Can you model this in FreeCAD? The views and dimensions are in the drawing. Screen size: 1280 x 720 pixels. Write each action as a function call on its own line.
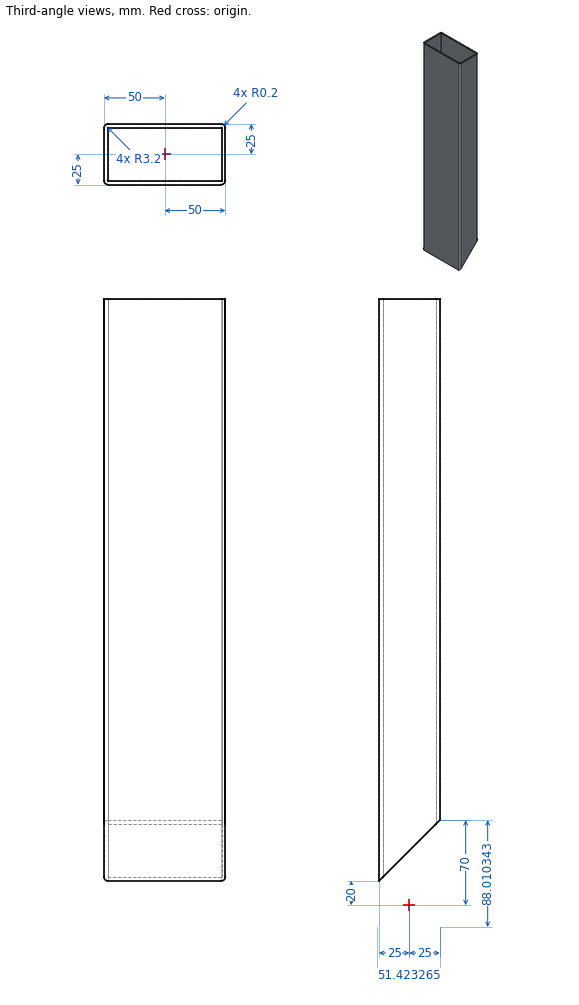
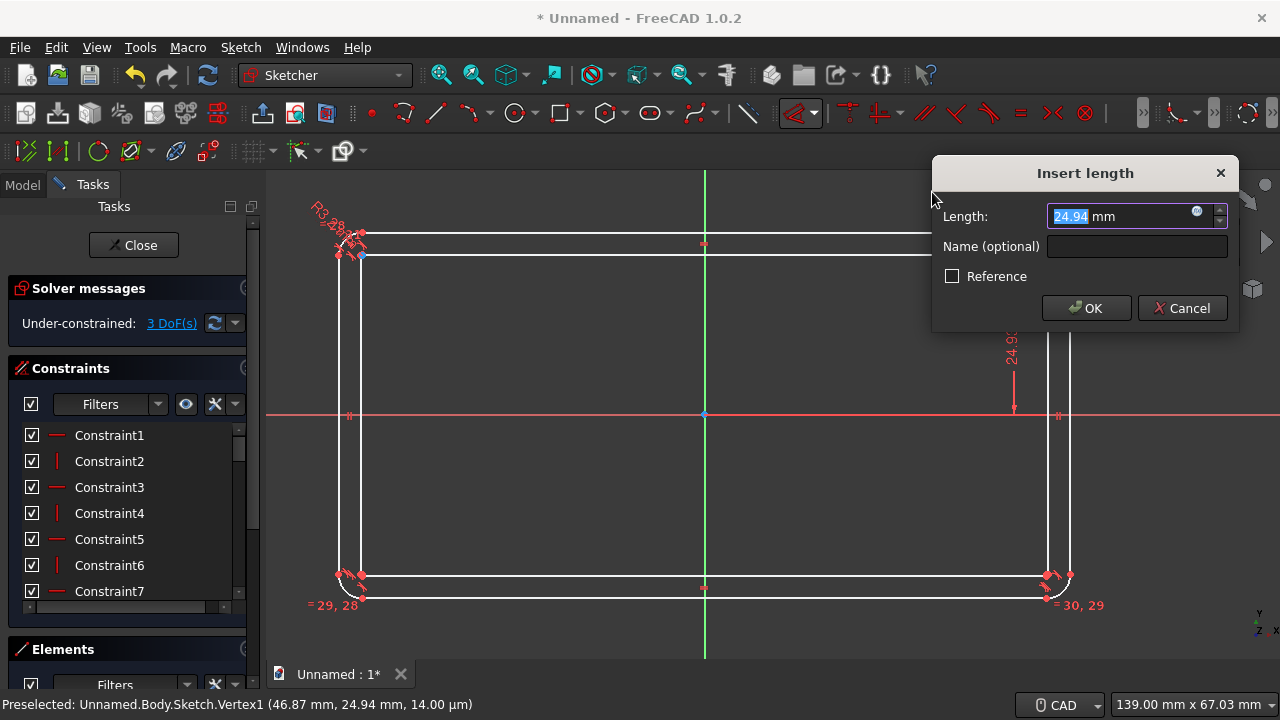
text(25)
key(Return)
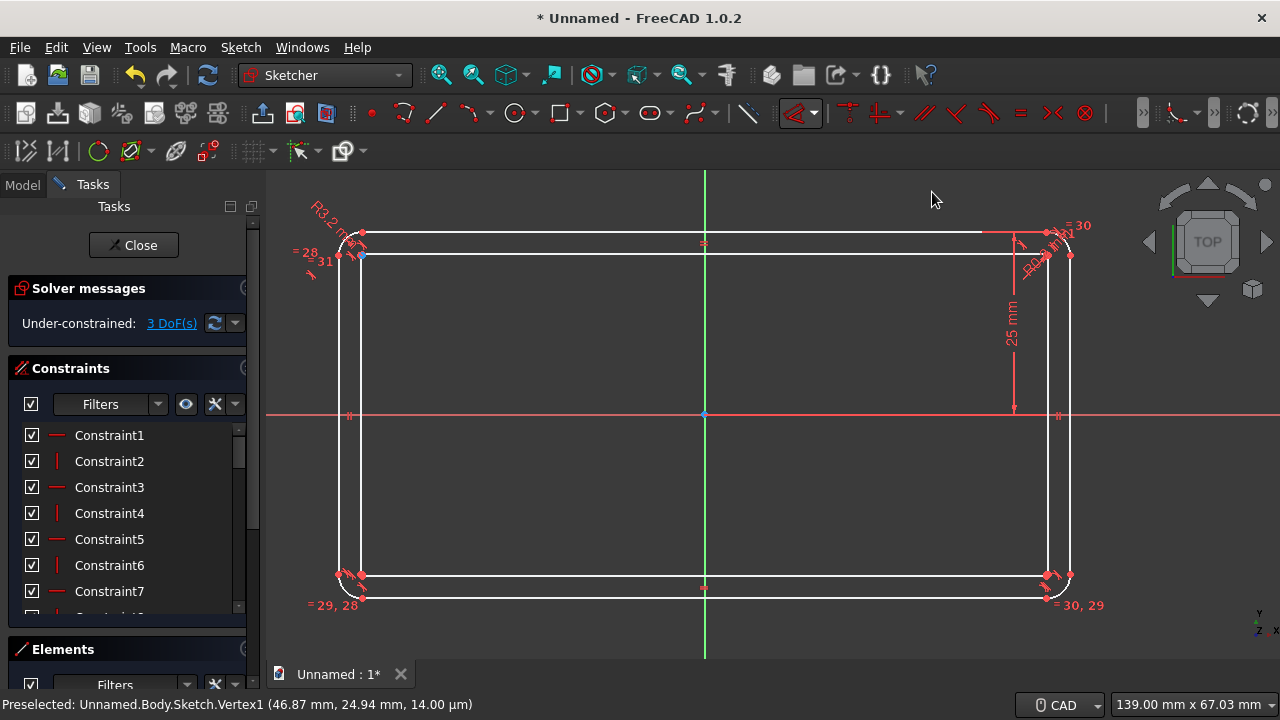
click(339, 256)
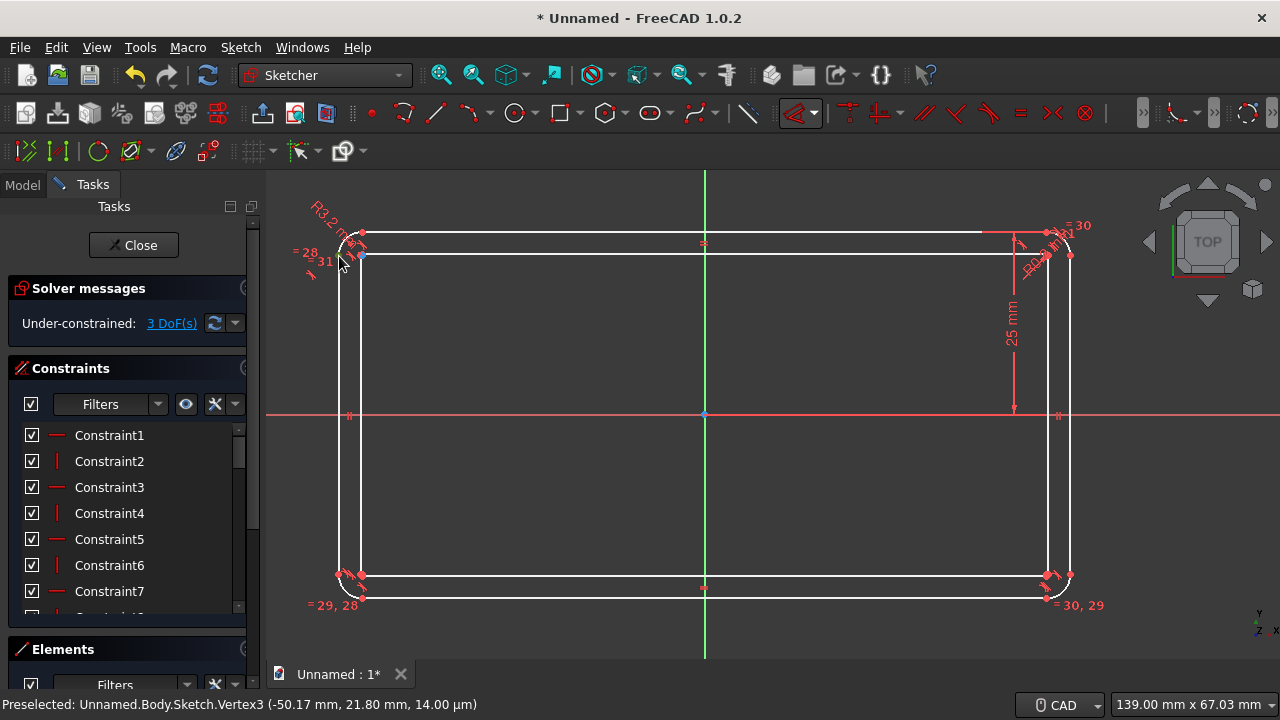
key(l)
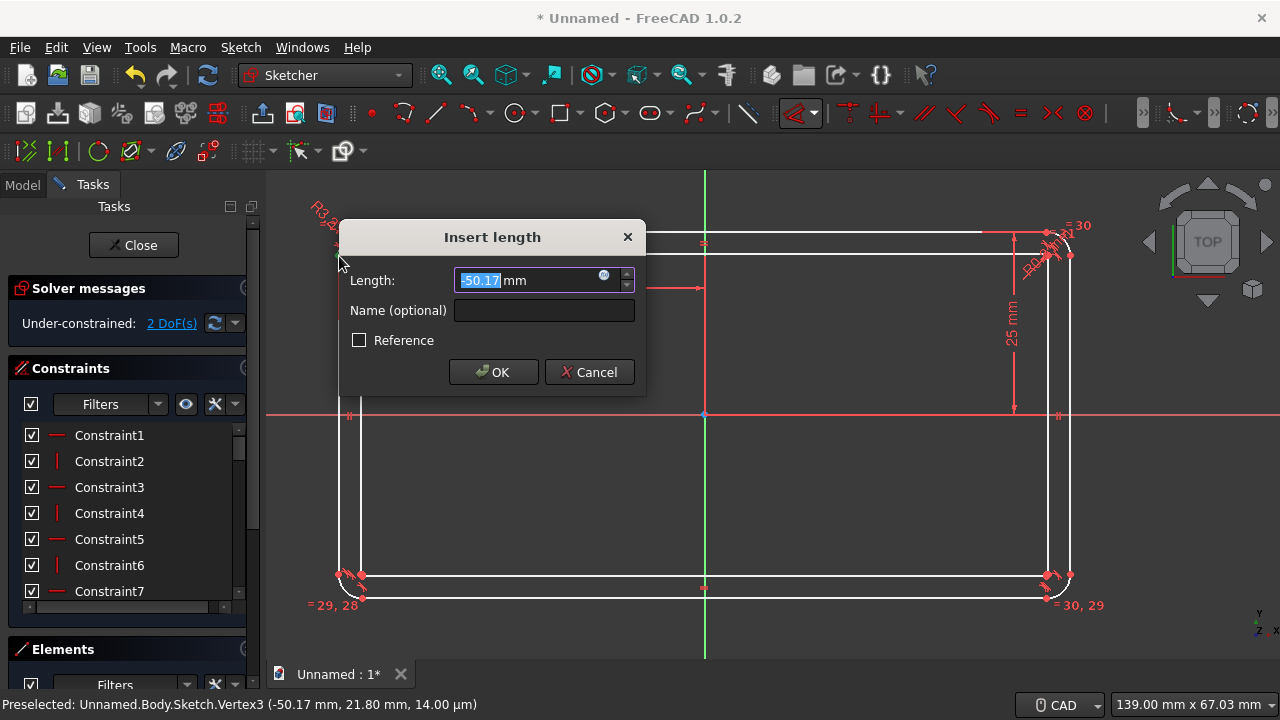
text(-50)
key(Return)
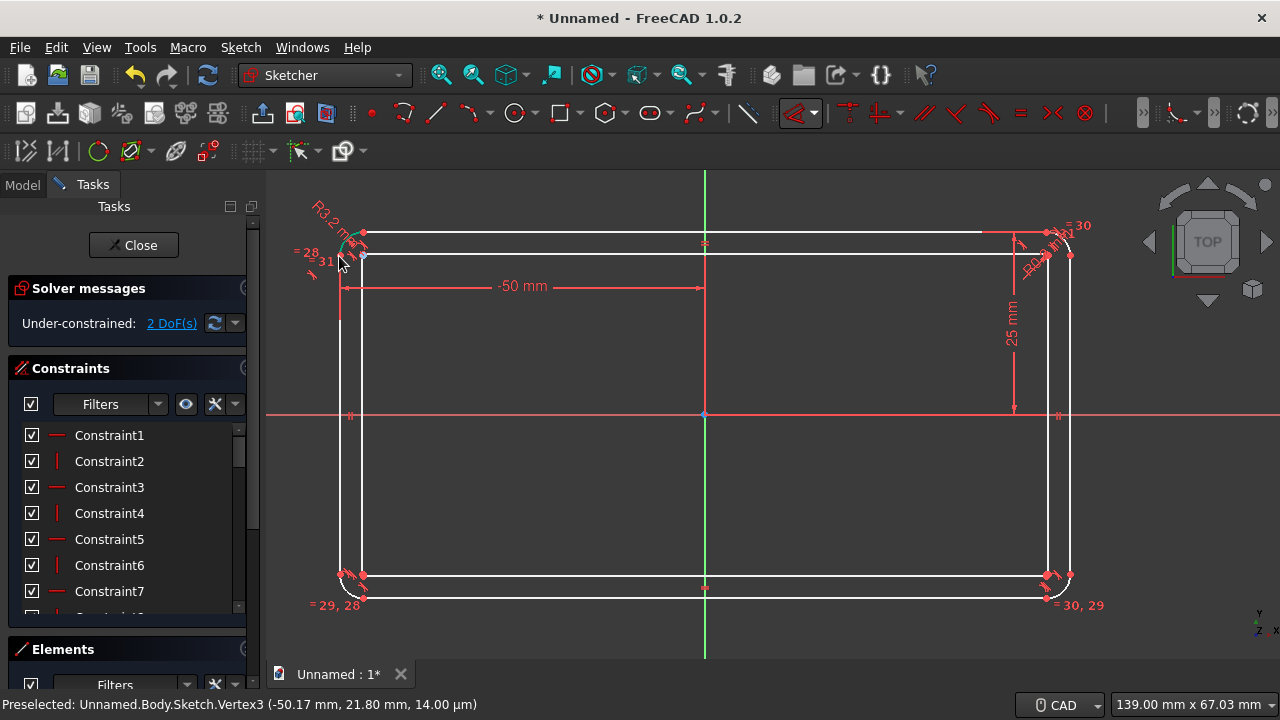
click(364, 598)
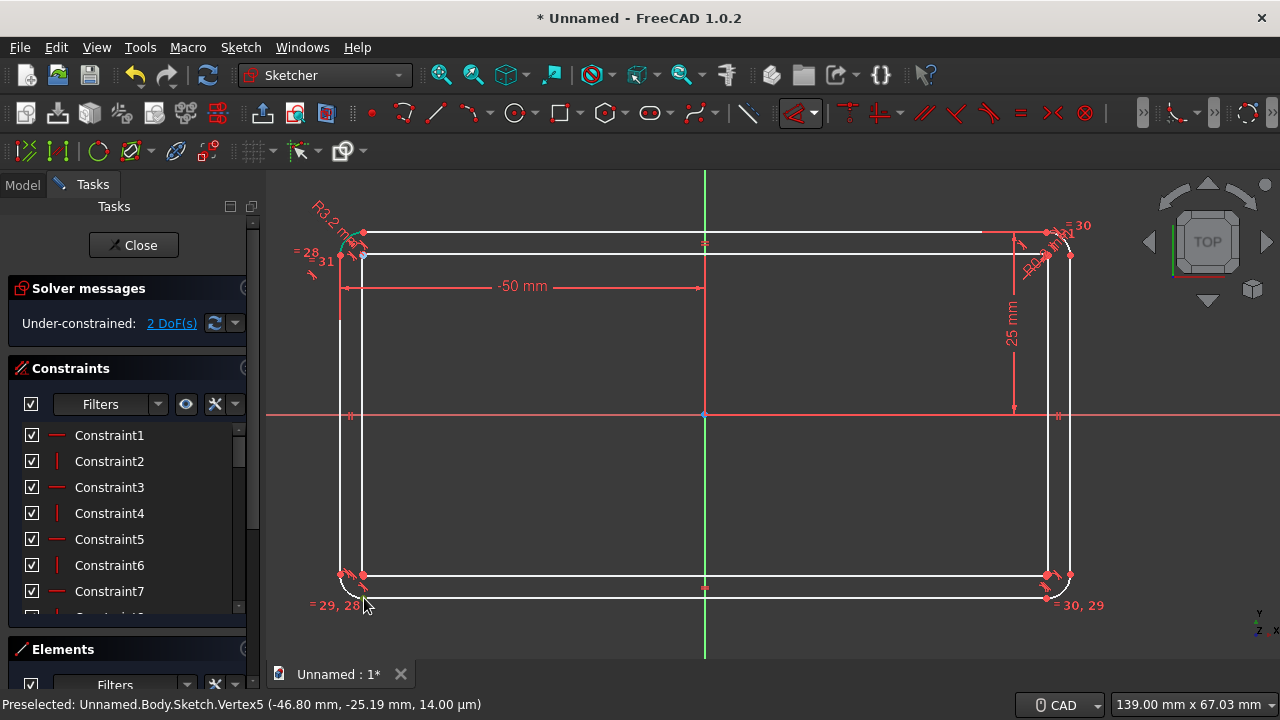
click(816, 114)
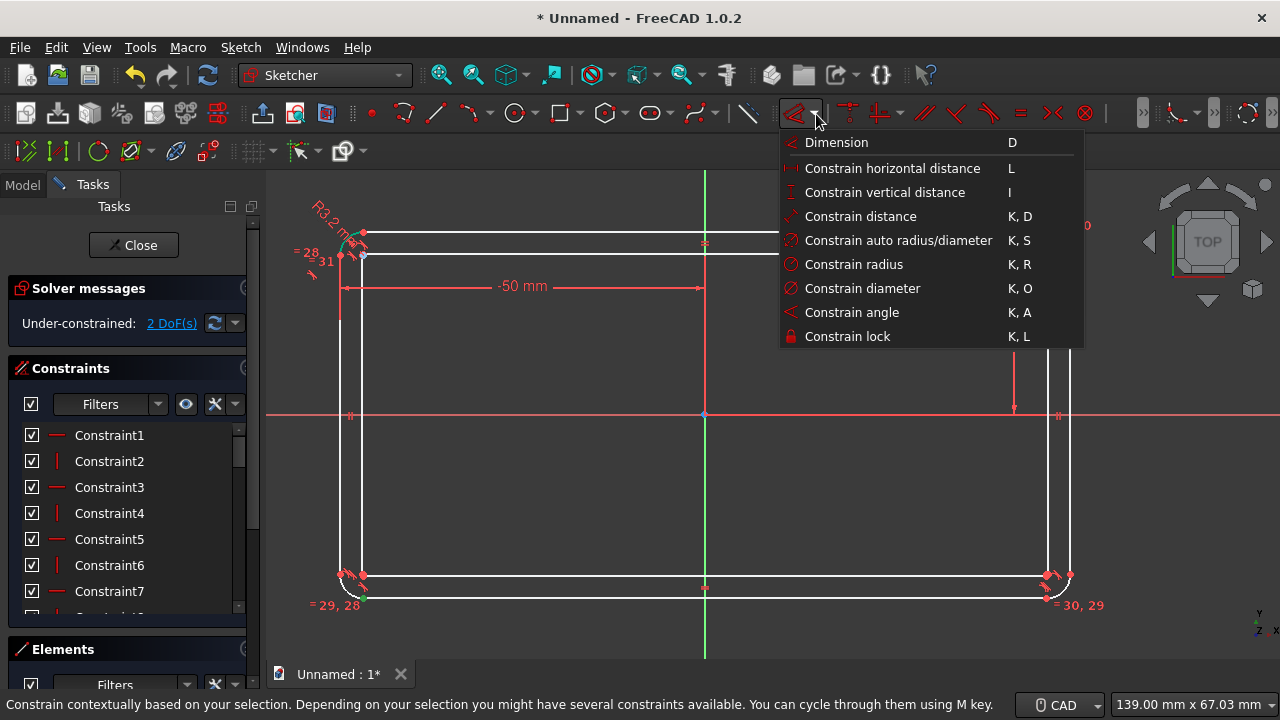
click(932, 192)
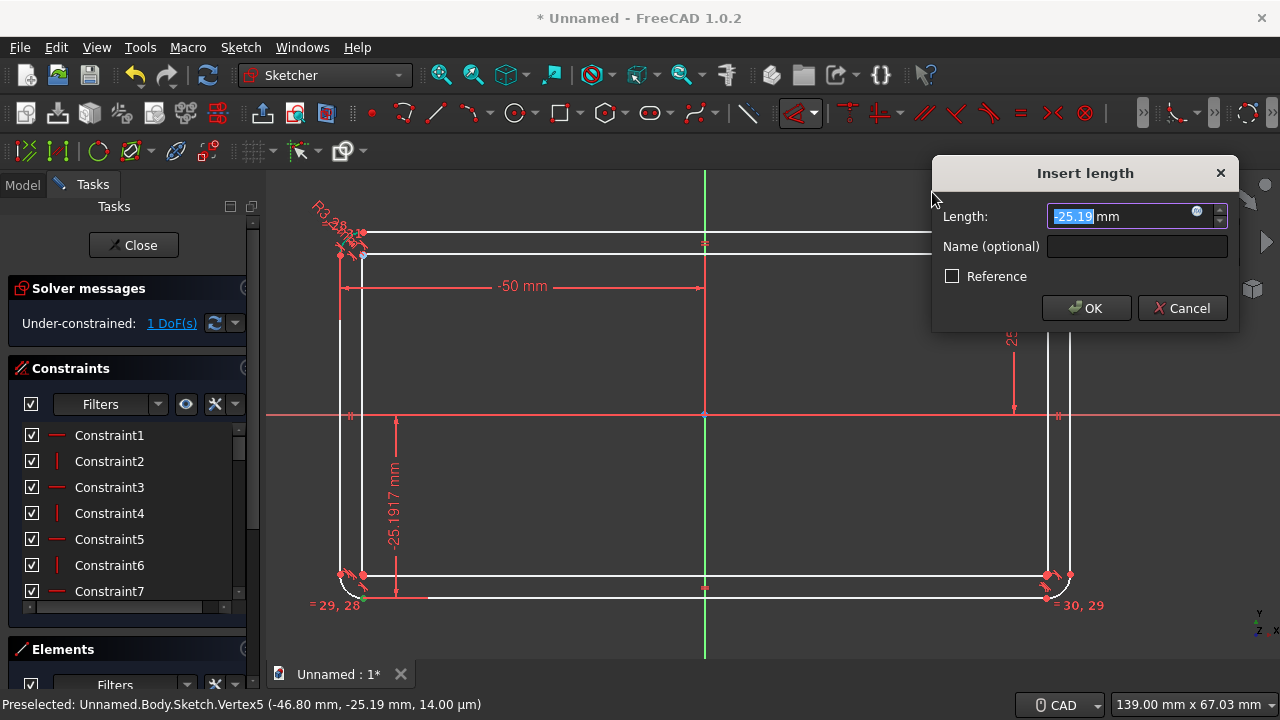
text(-25)
key(Return)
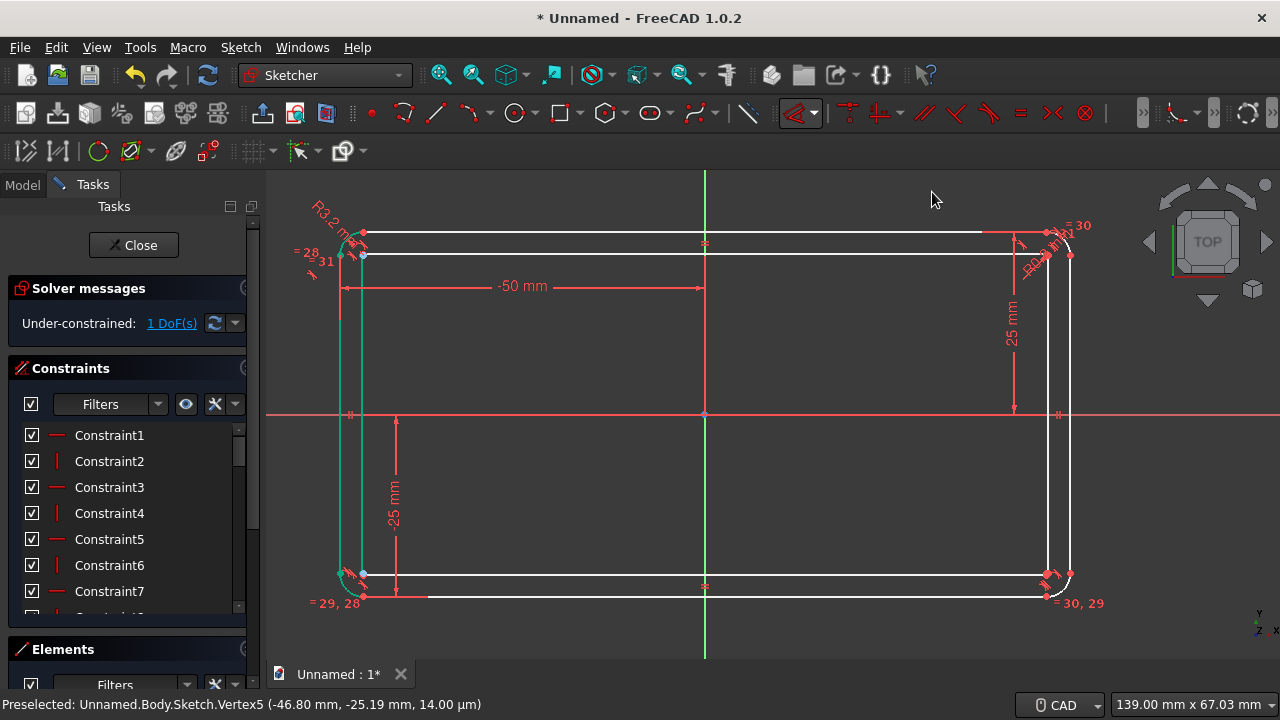
click(1070, 574)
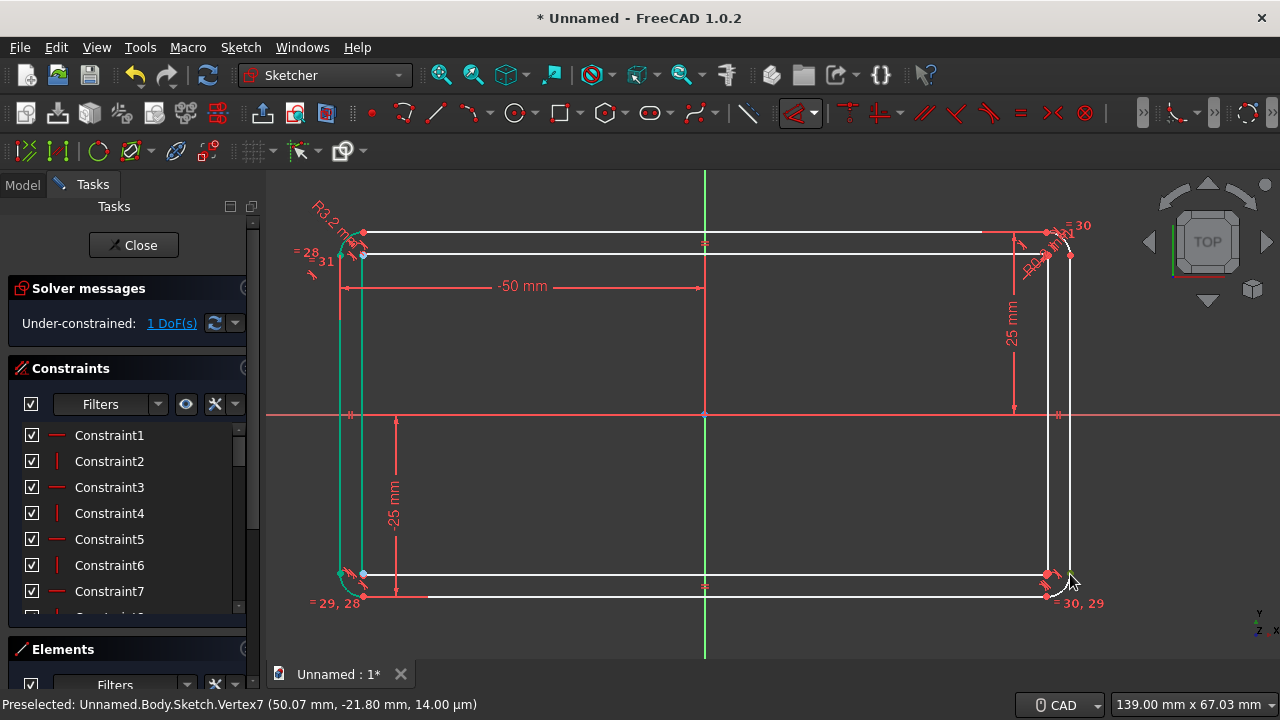
click(816, 114)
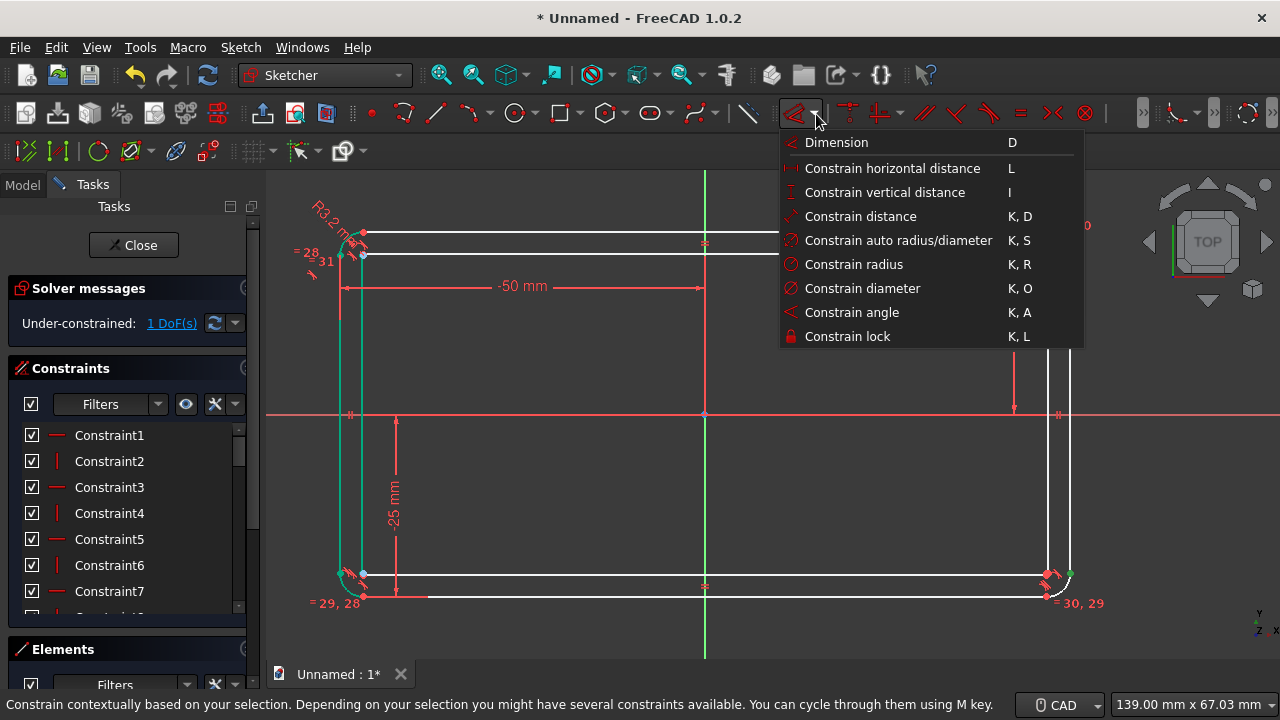
click(932, 168)